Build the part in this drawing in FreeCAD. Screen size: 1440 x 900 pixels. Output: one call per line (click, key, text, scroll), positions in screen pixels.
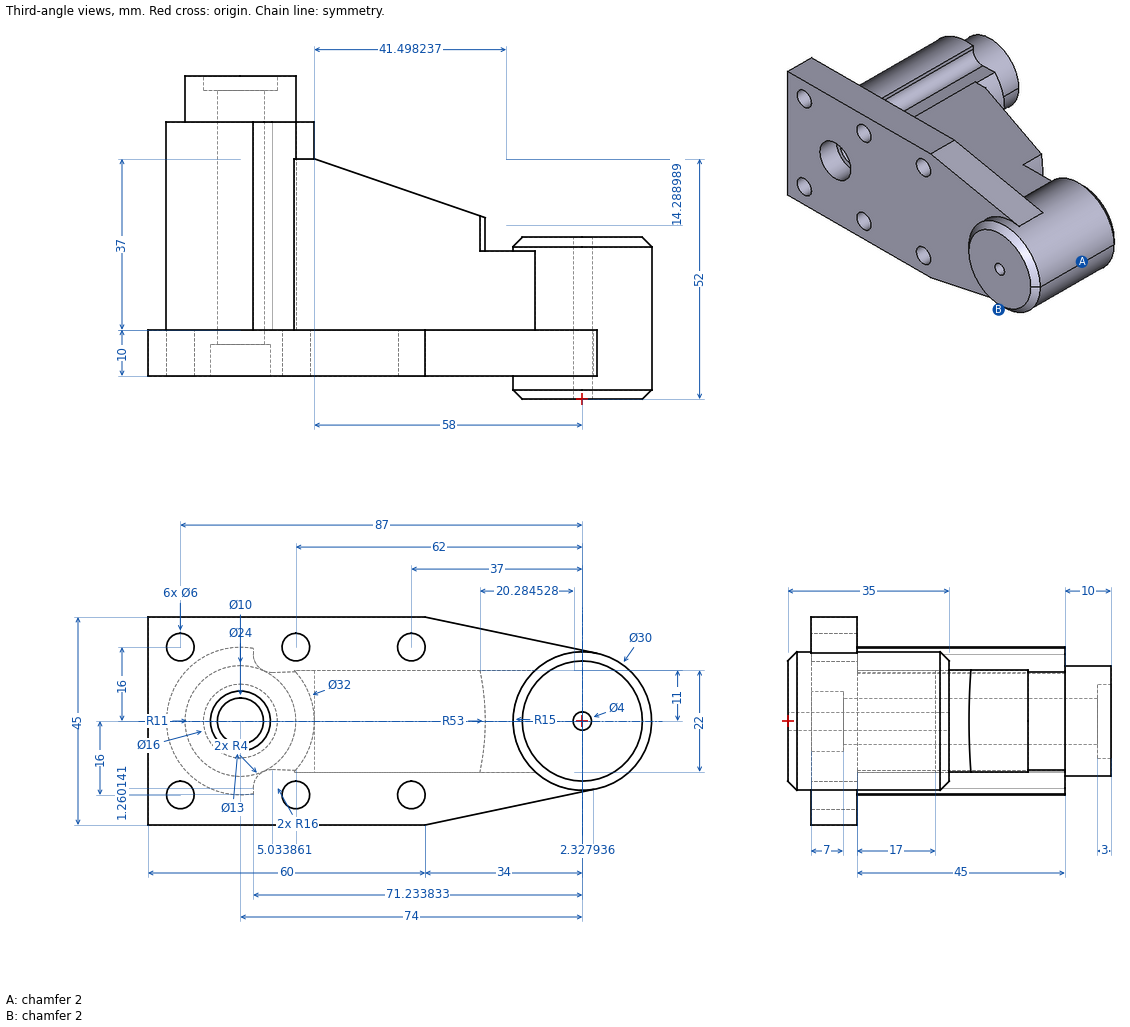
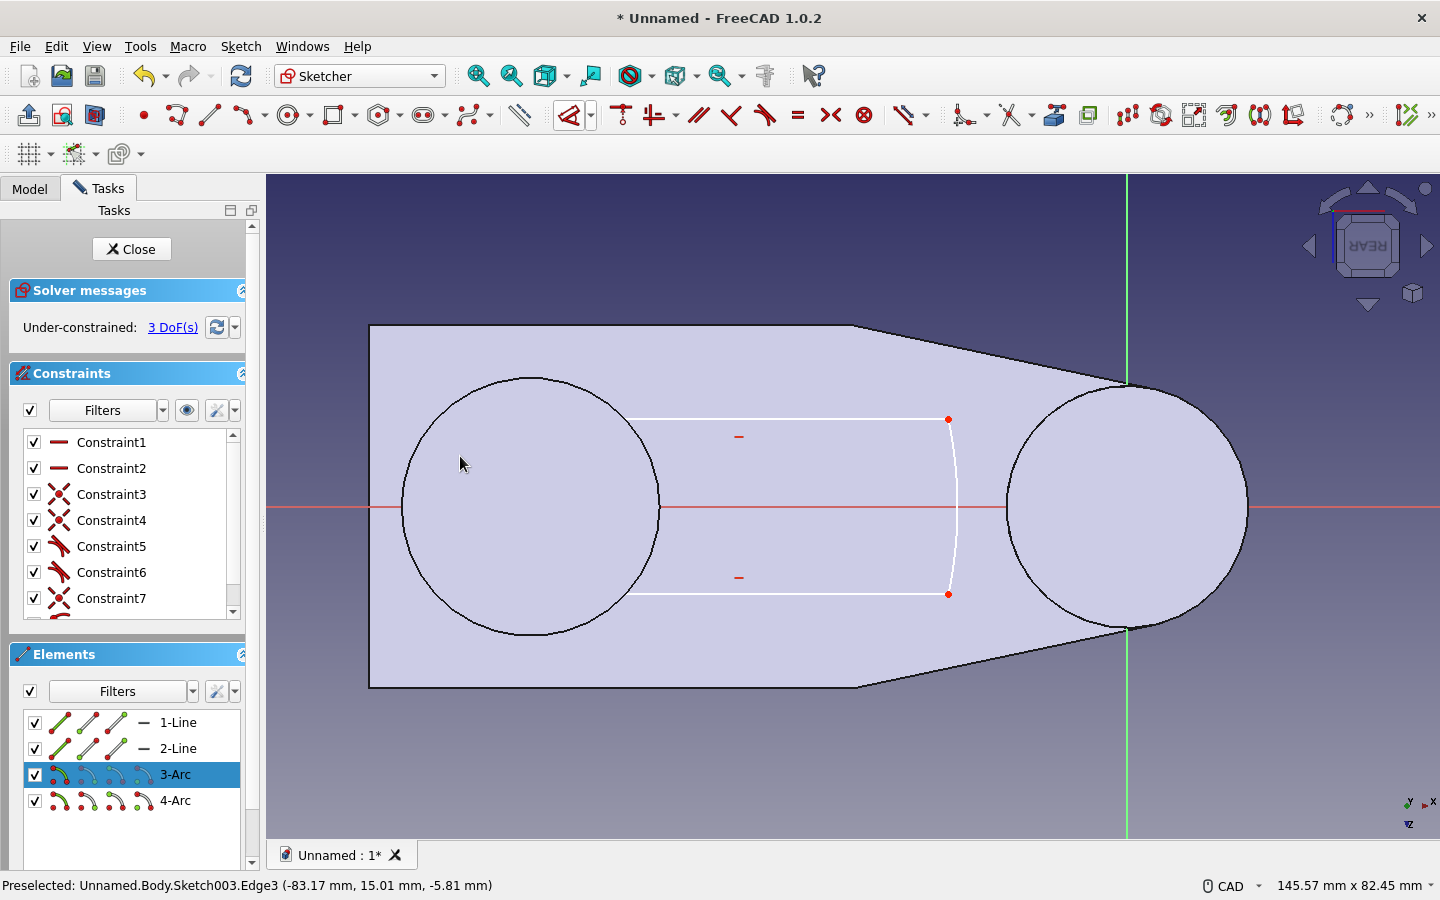
key(k)
key(r)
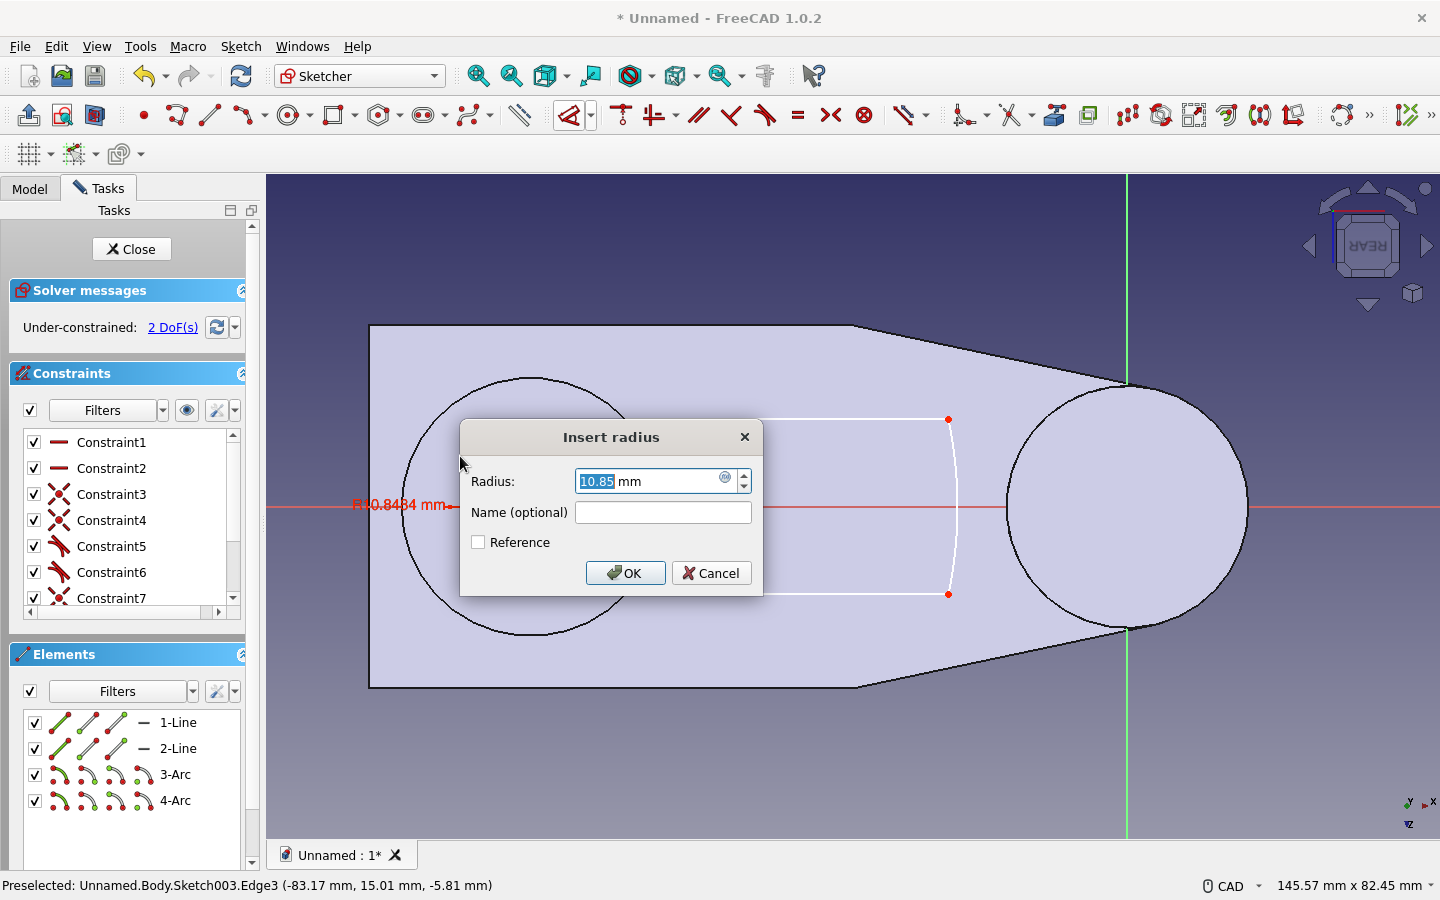
text(11)
key(Return)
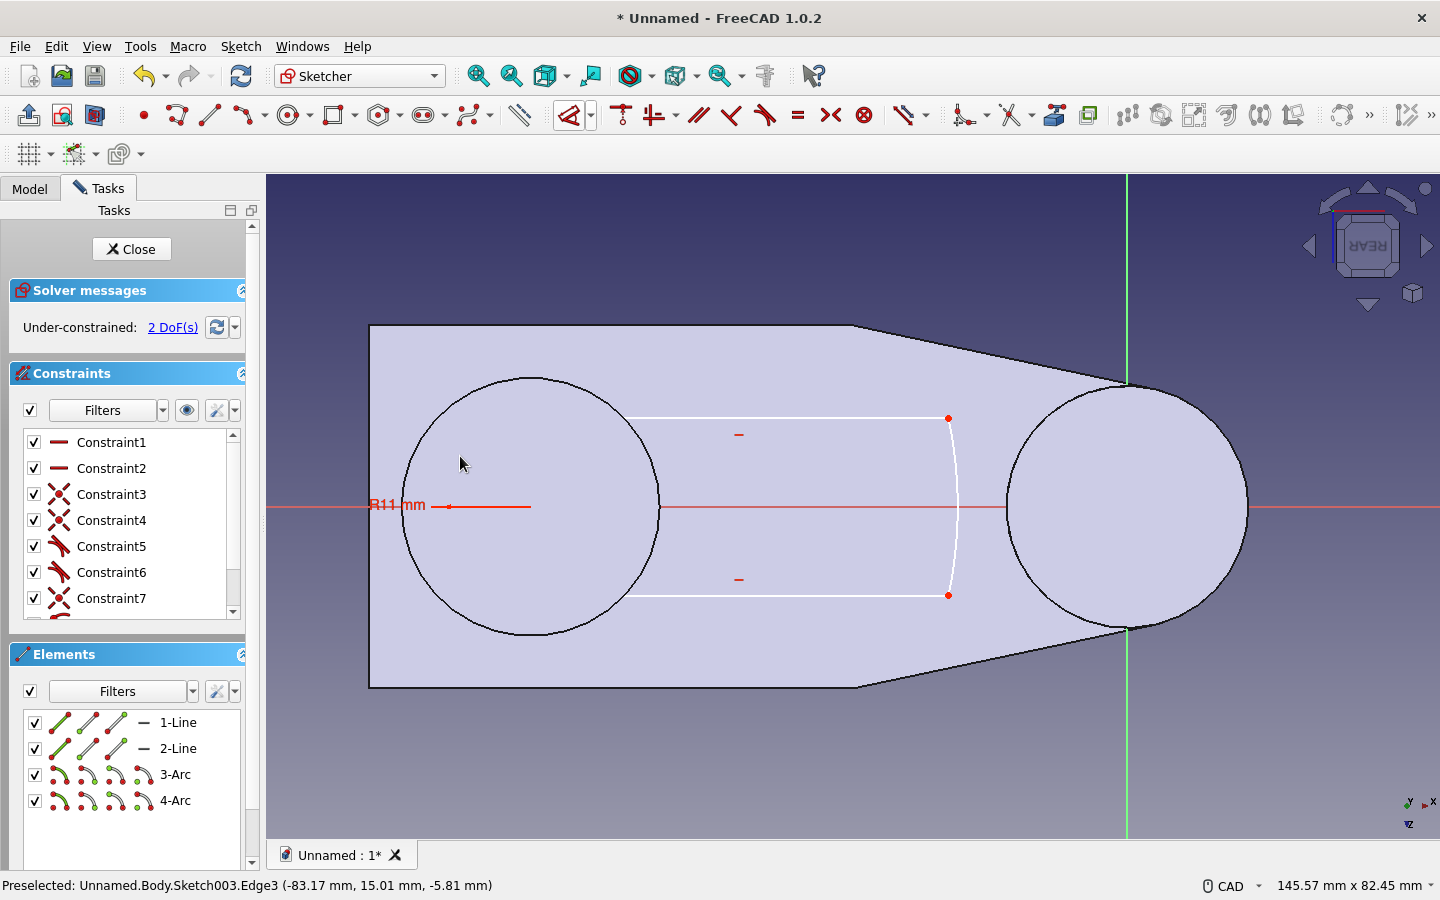
click(956, 543)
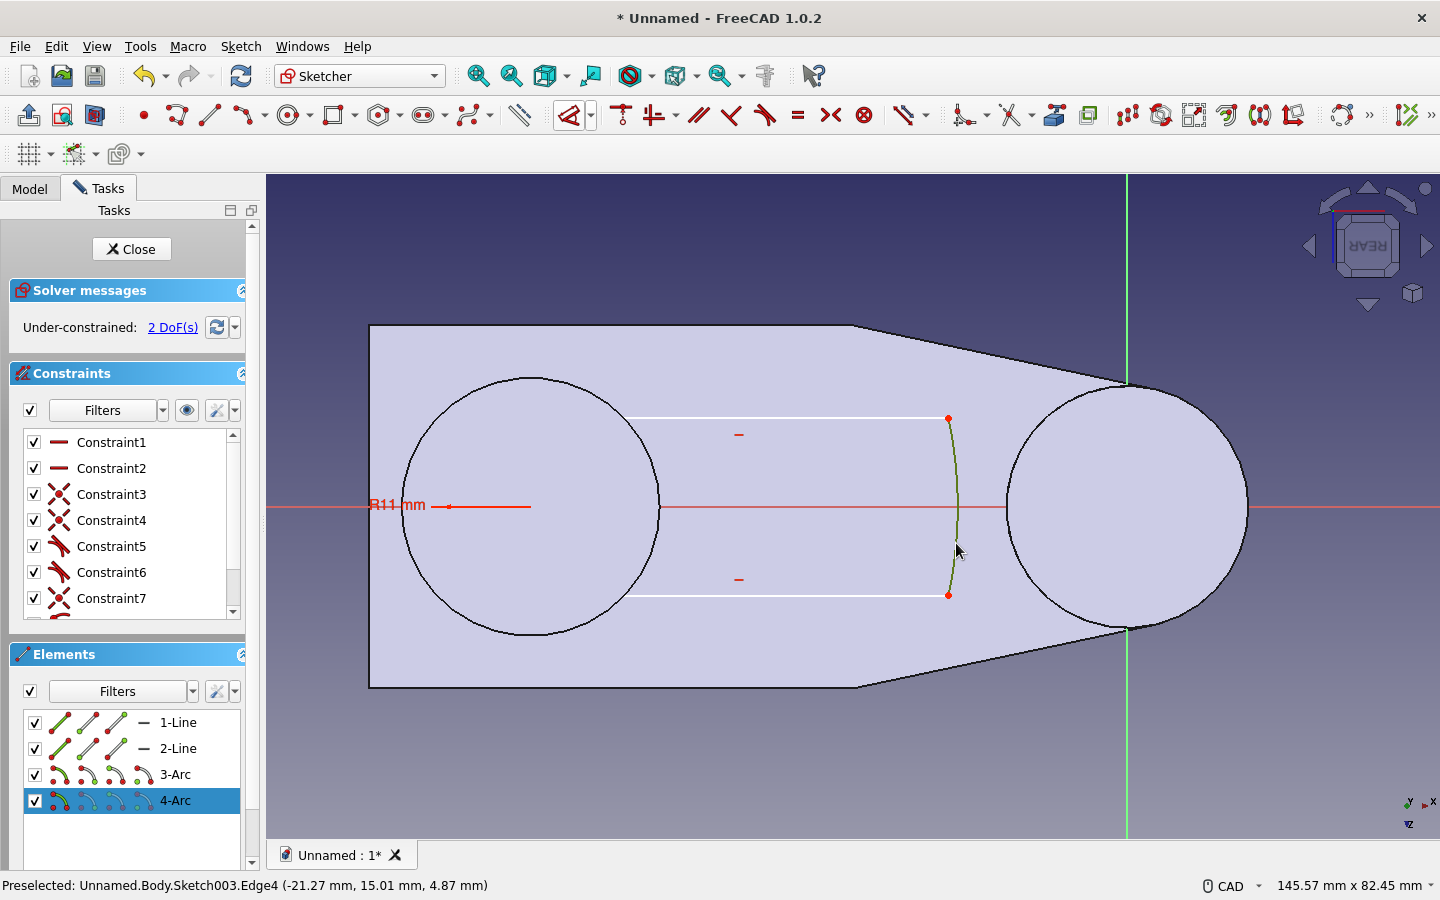
click(590, 116)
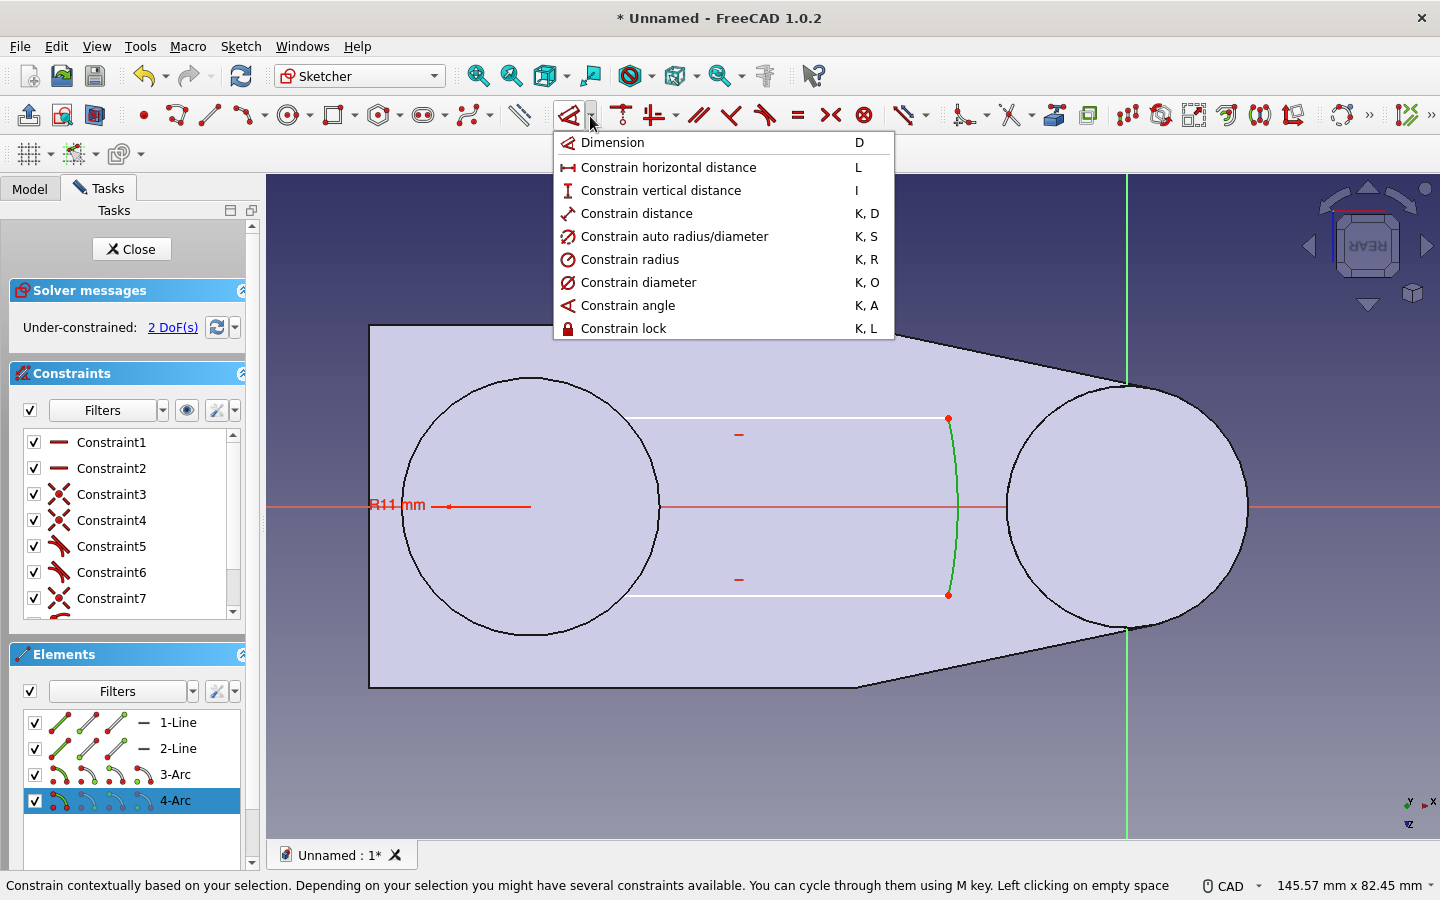
click(724, 260)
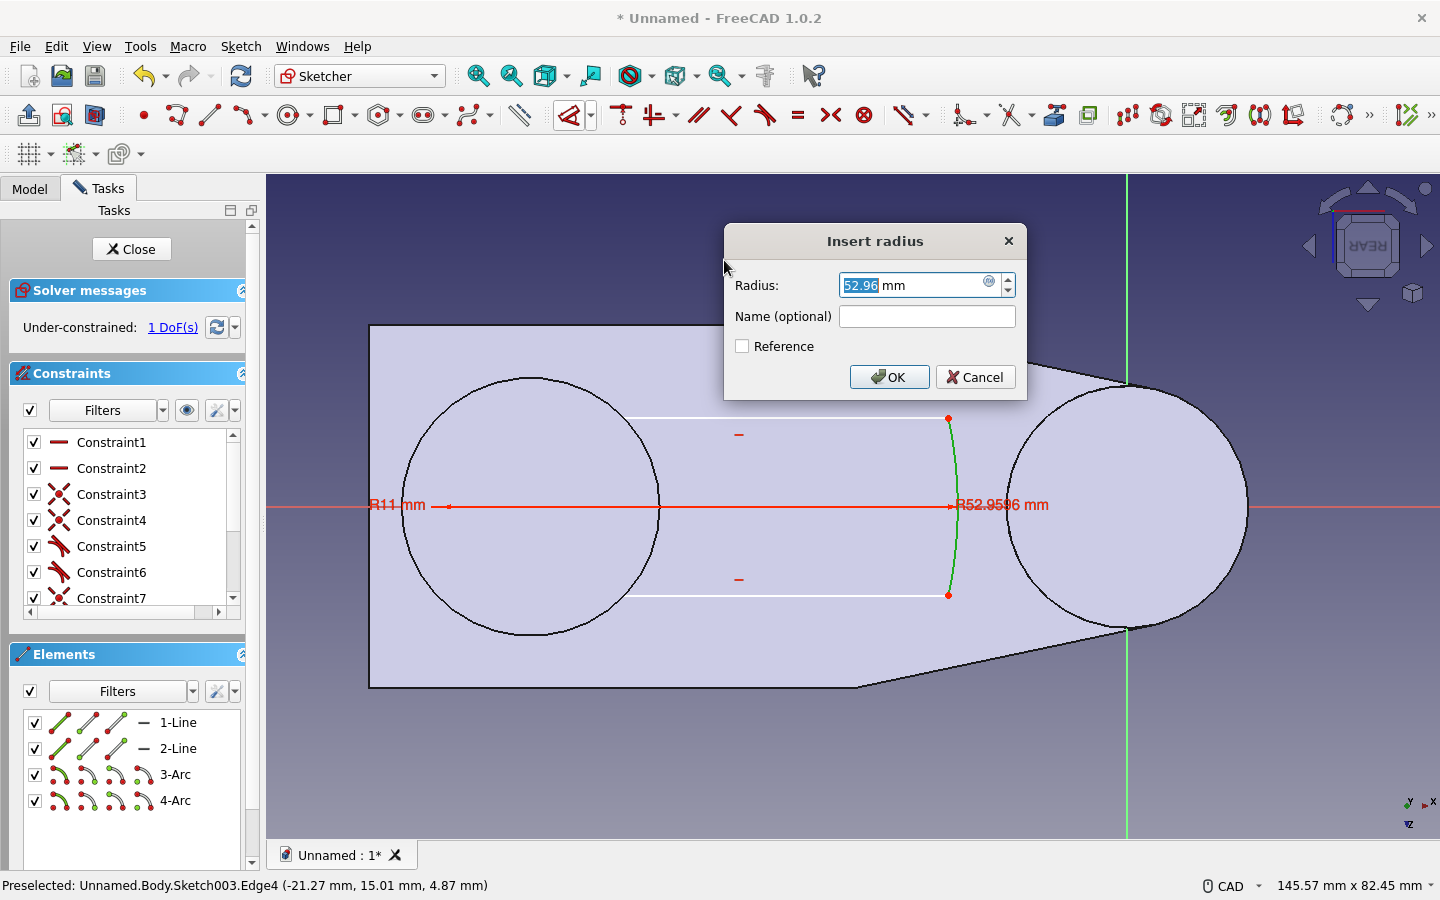
text(53)
key(Return)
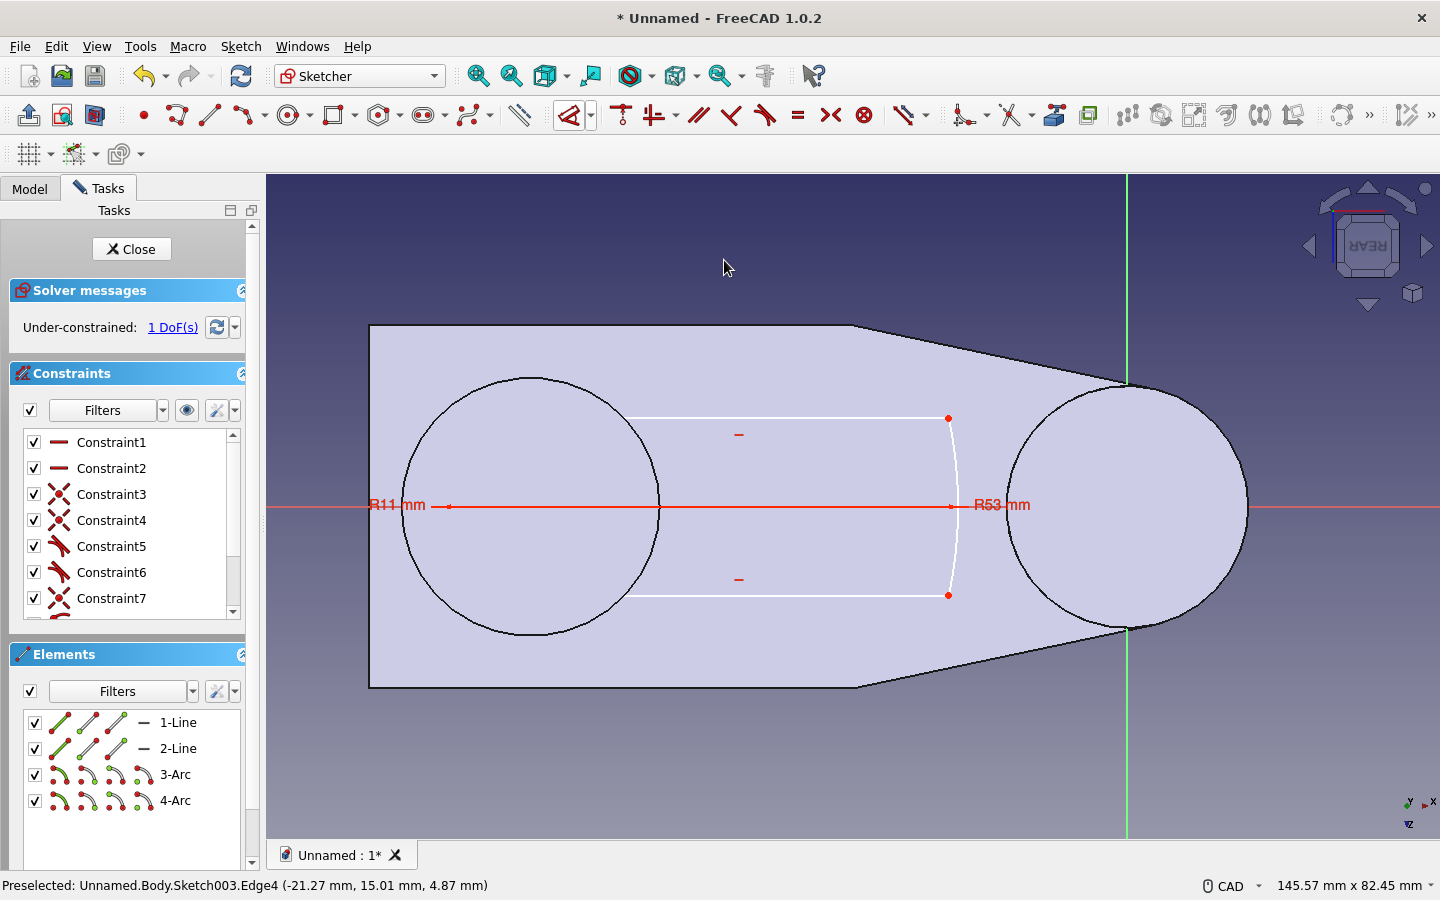
click(531, 418)